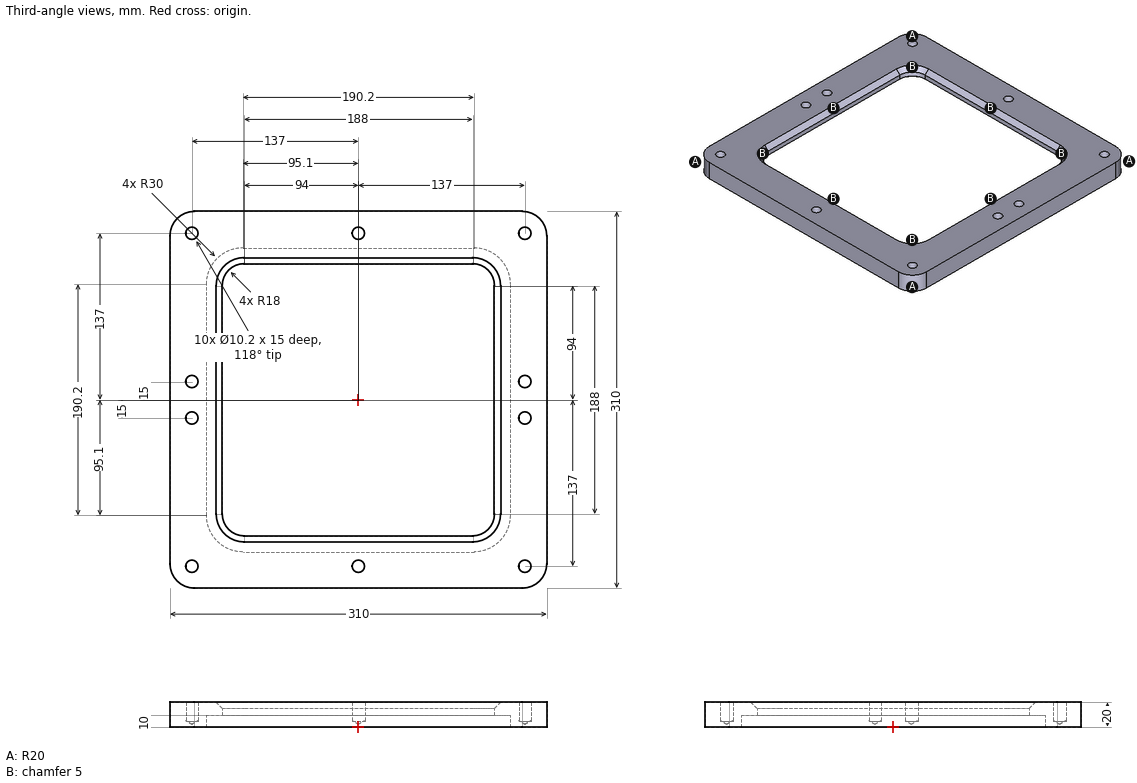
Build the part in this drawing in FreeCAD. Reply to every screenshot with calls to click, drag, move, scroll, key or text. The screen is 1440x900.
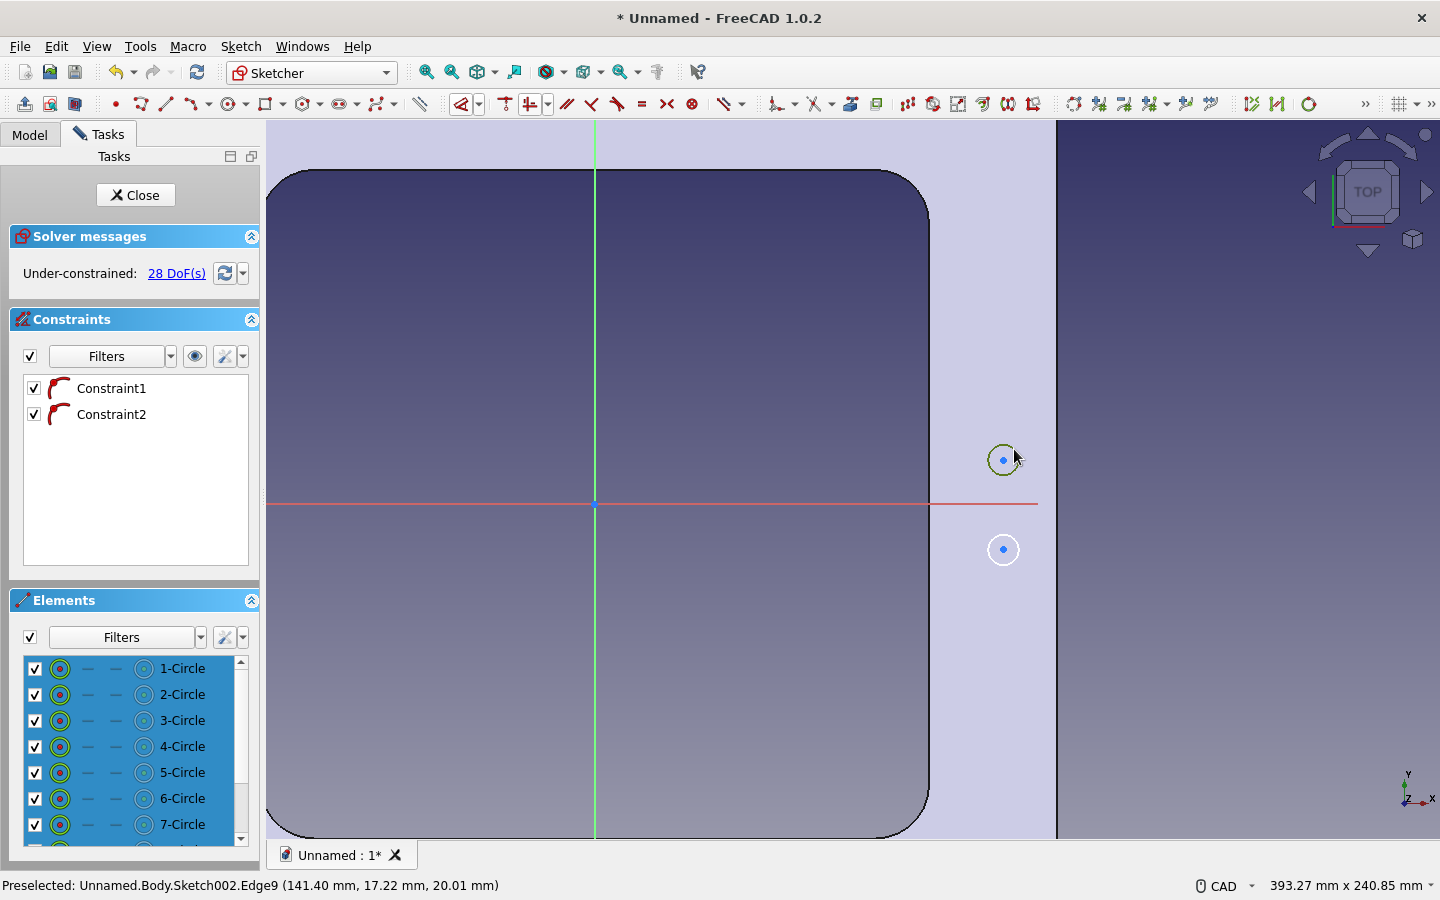
click(1014, 539)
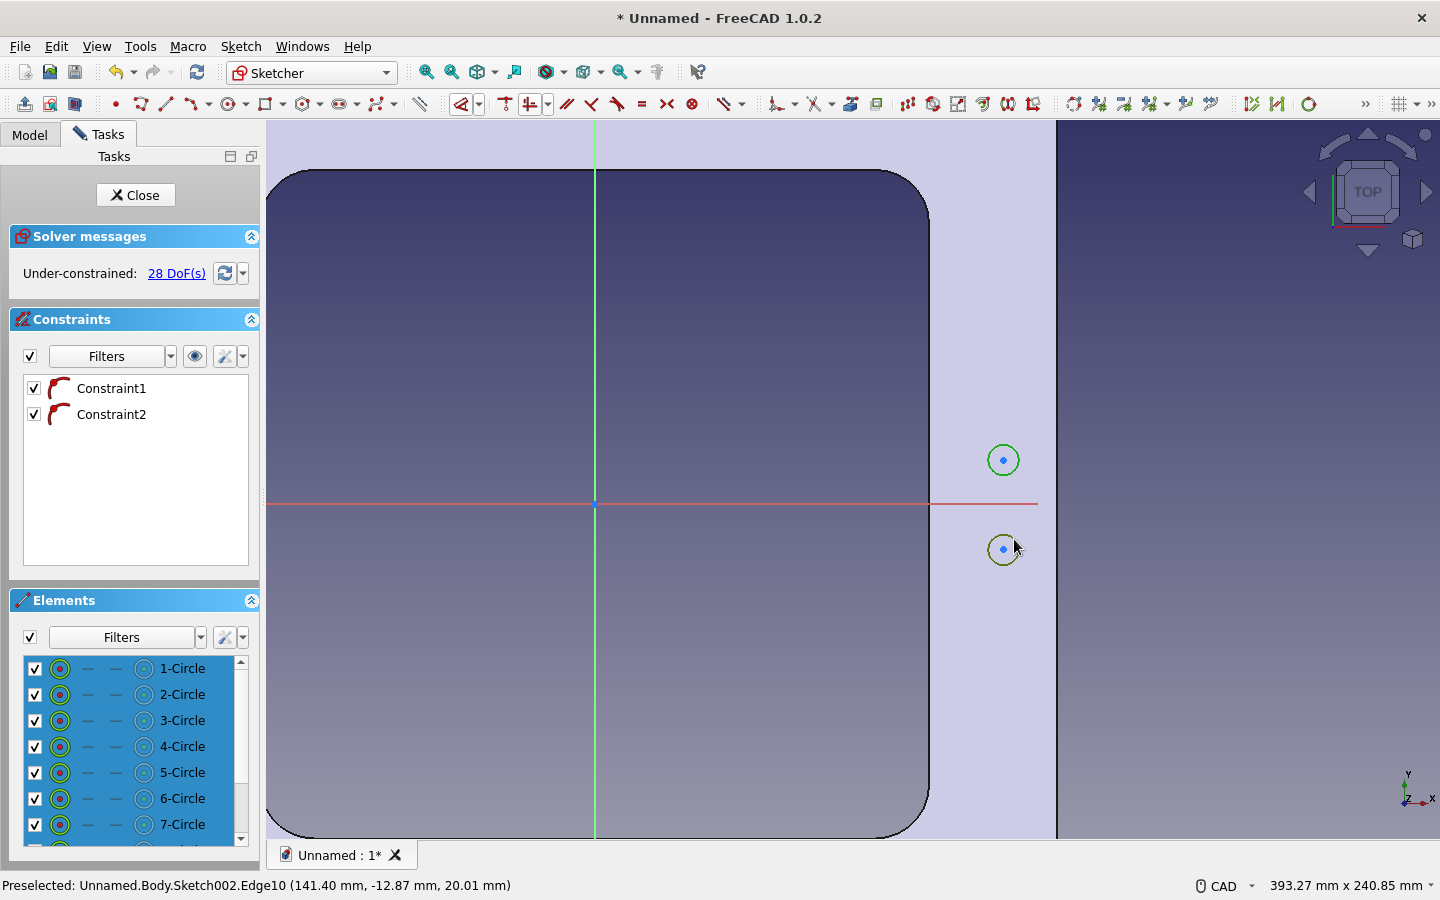
click(642, 104)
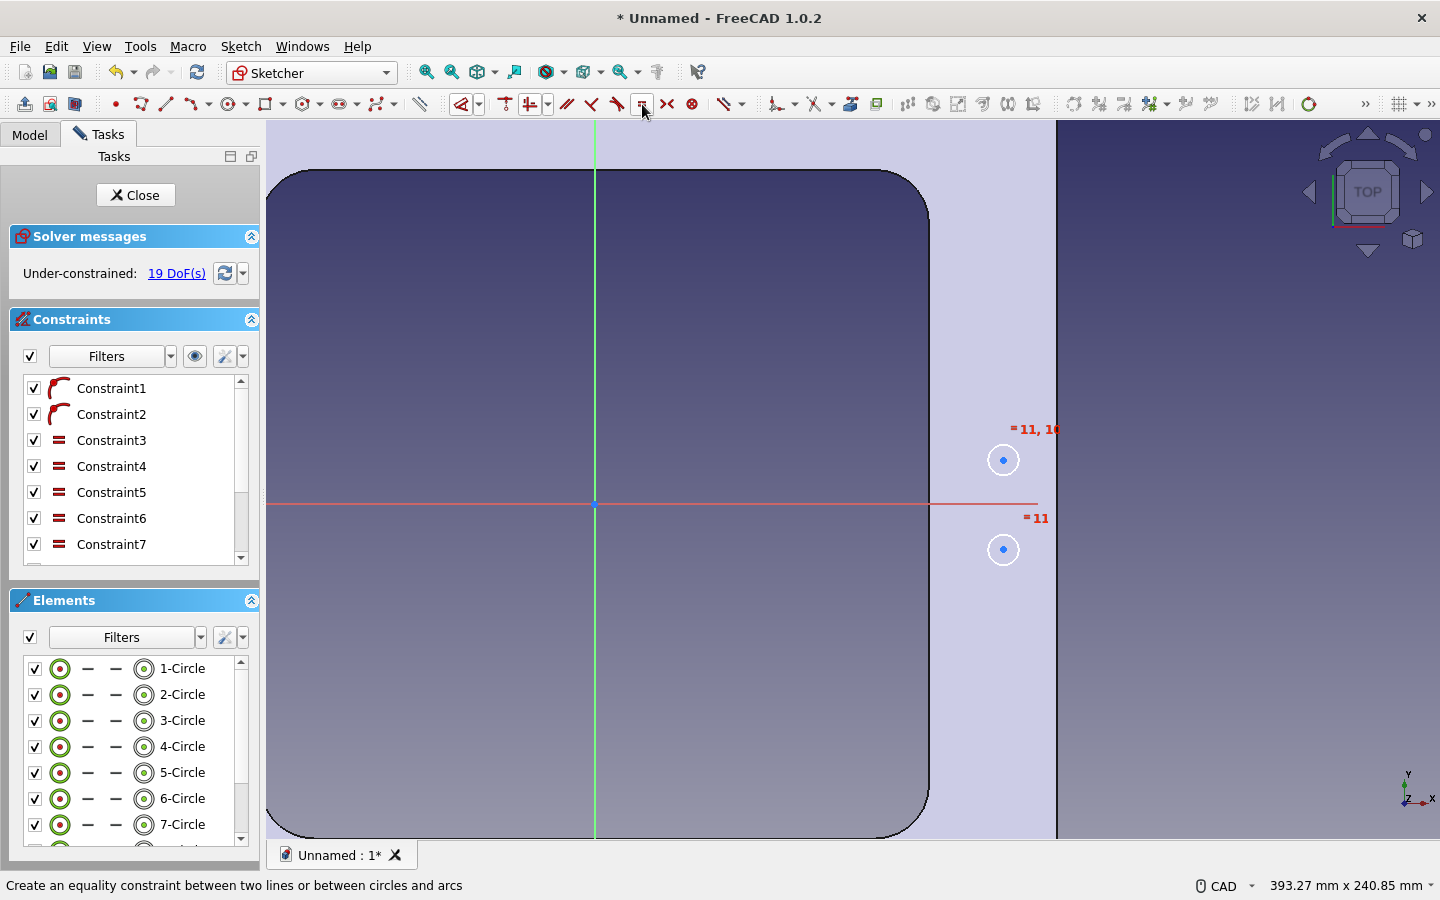
scroll(1015, 449, down, 3)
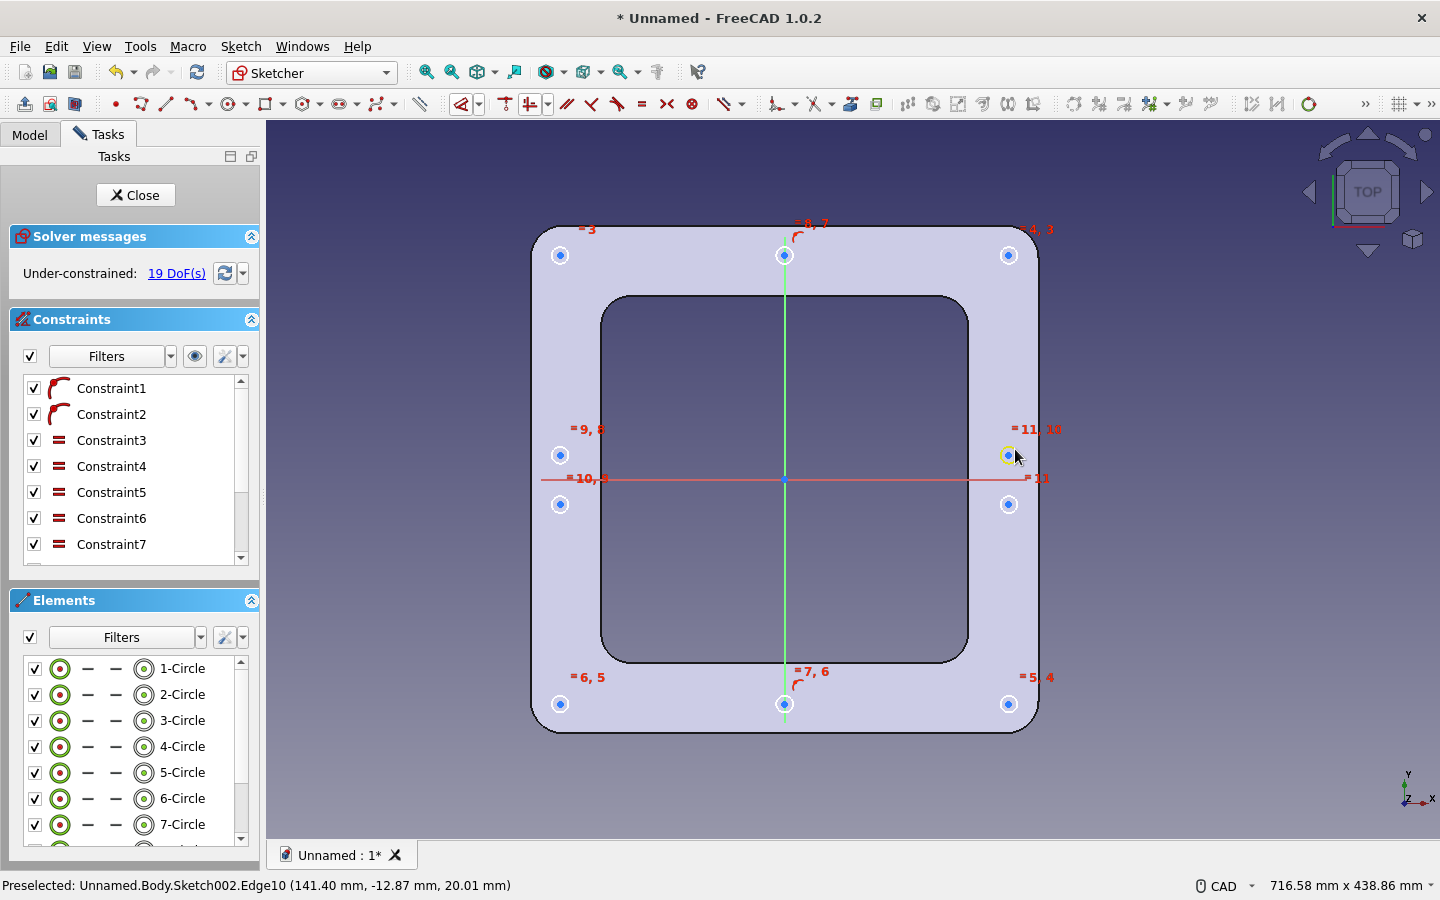
click(560, 255)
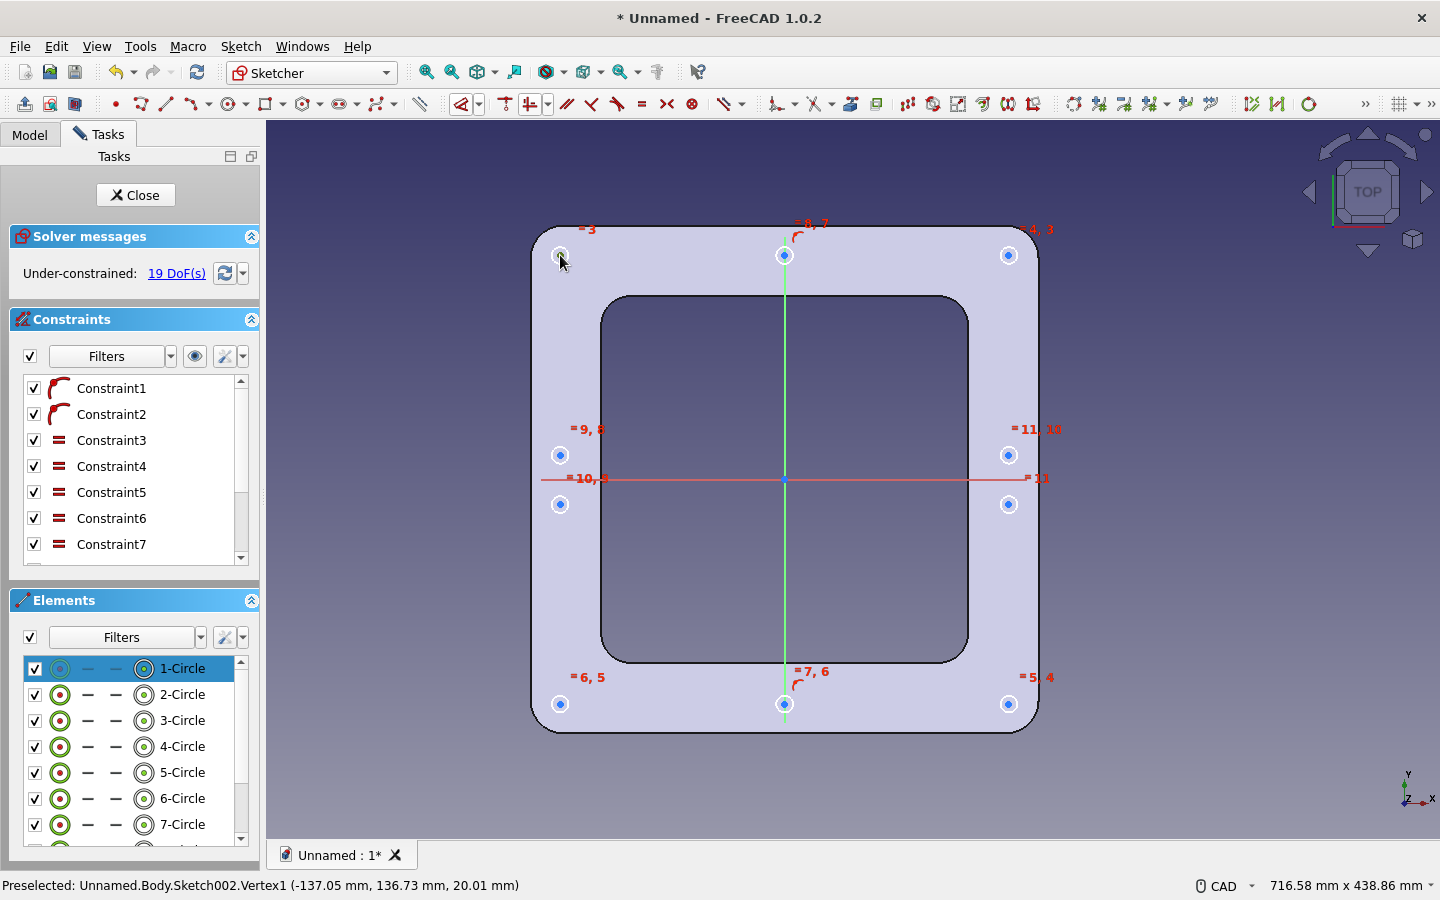
click(1009, 255)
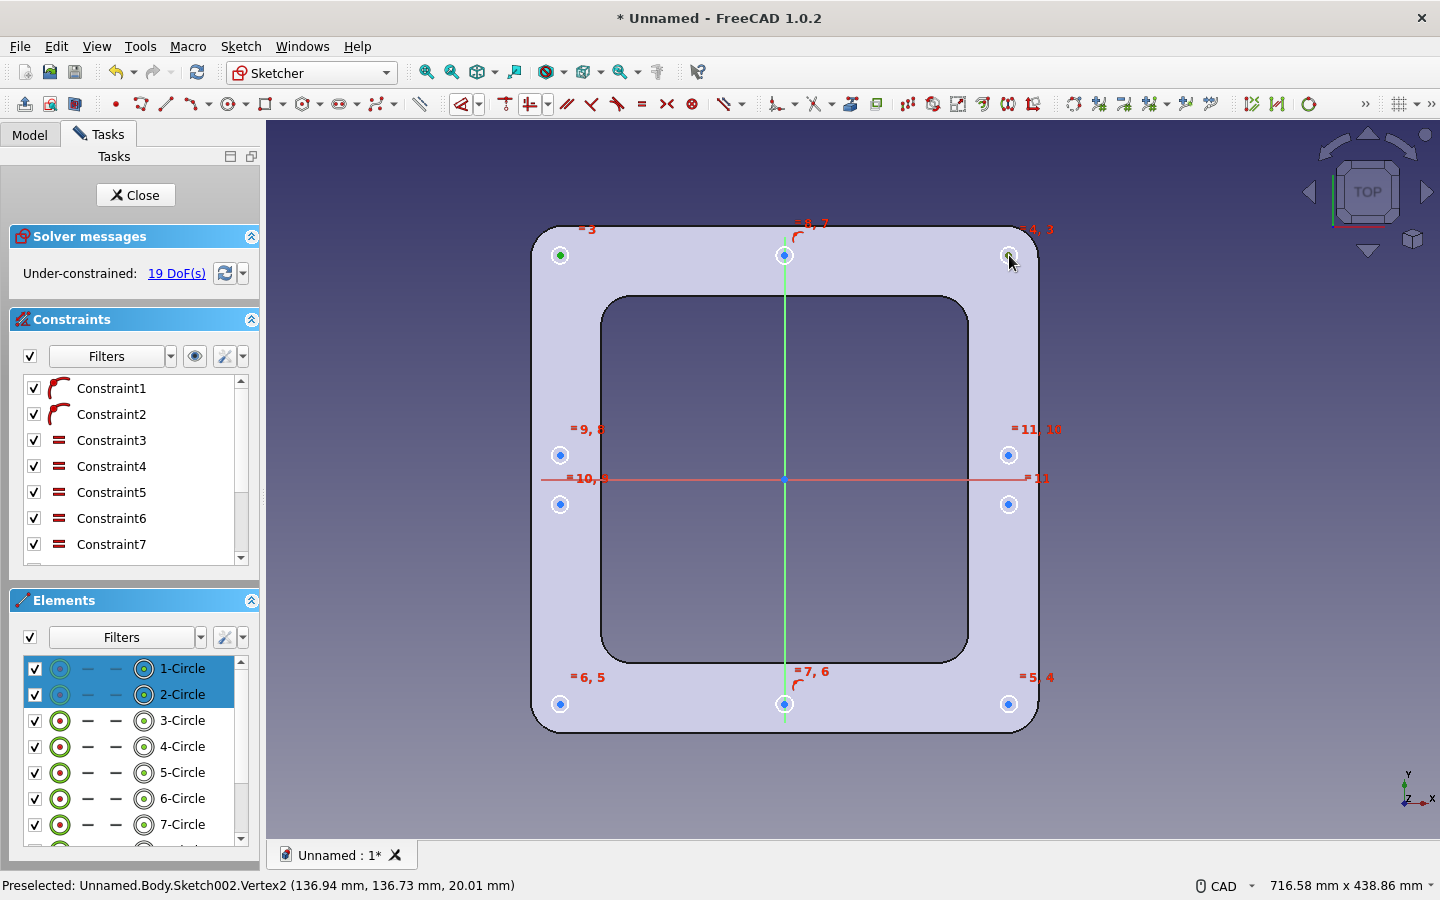
key(h)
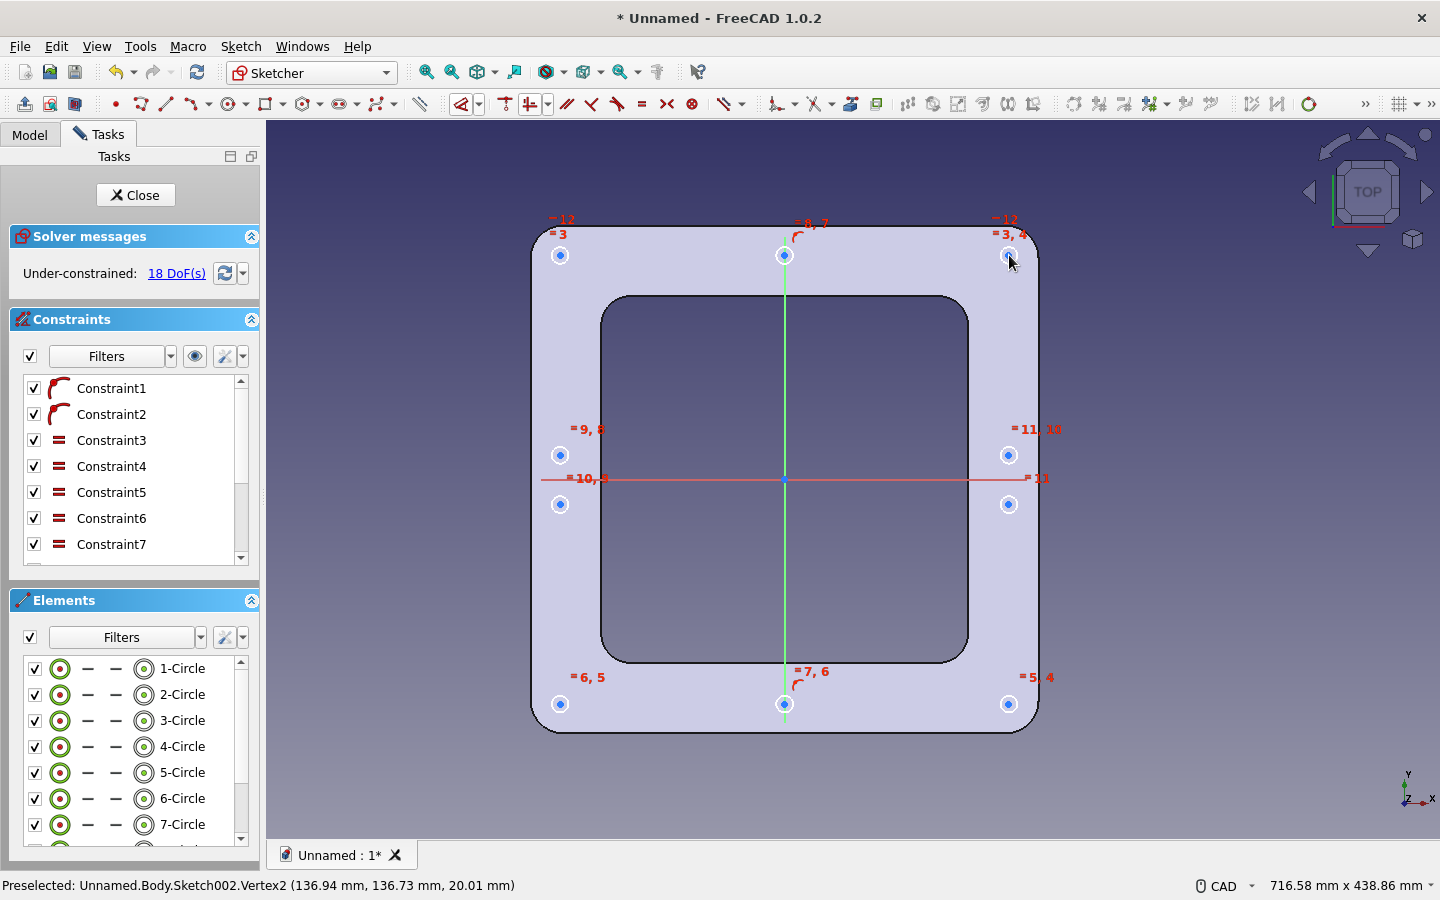
click(1009, 255)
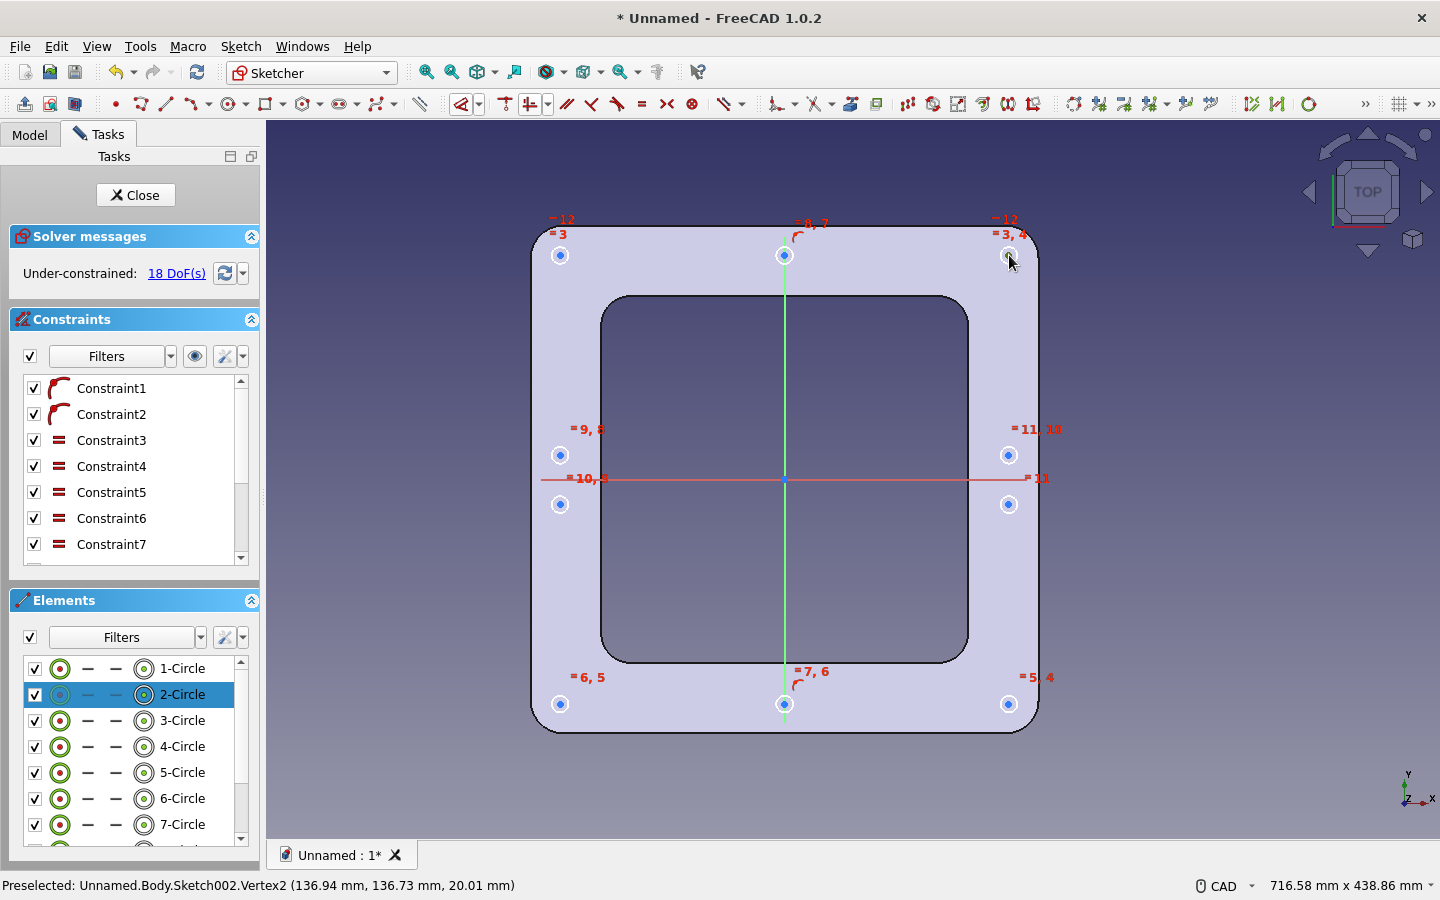
click(1009, 704)